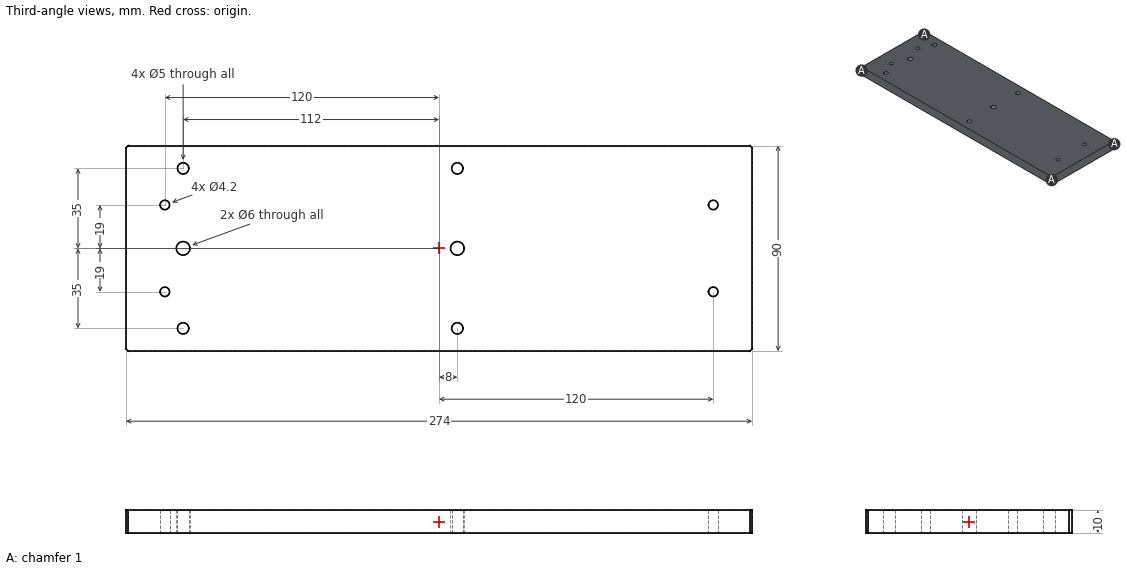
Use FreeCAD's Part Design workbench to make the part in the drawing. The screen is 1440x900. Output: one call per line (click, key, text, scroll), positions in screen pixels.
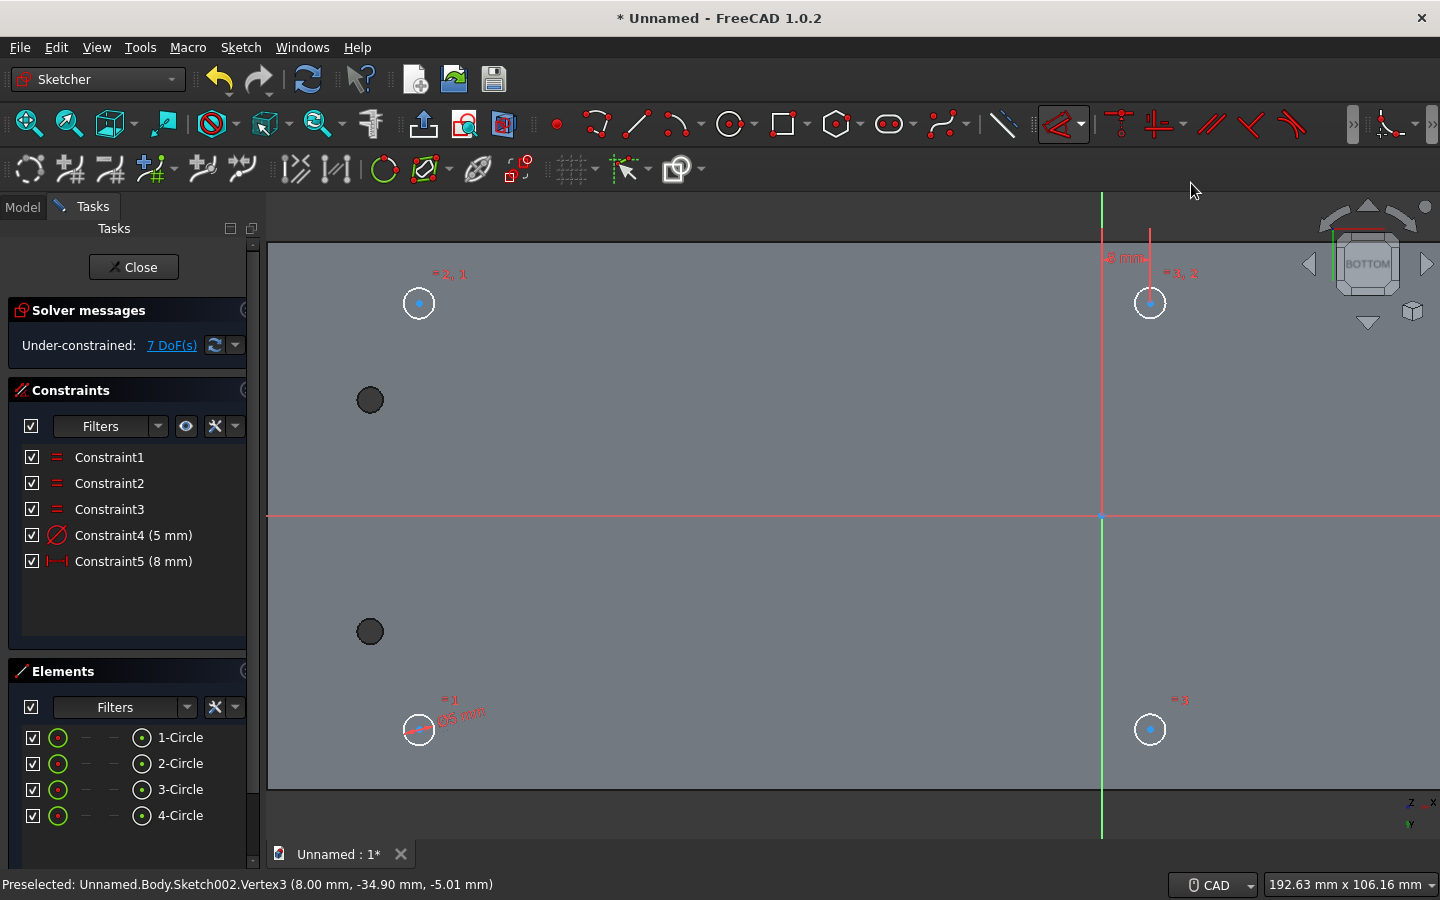
click(1150, 730)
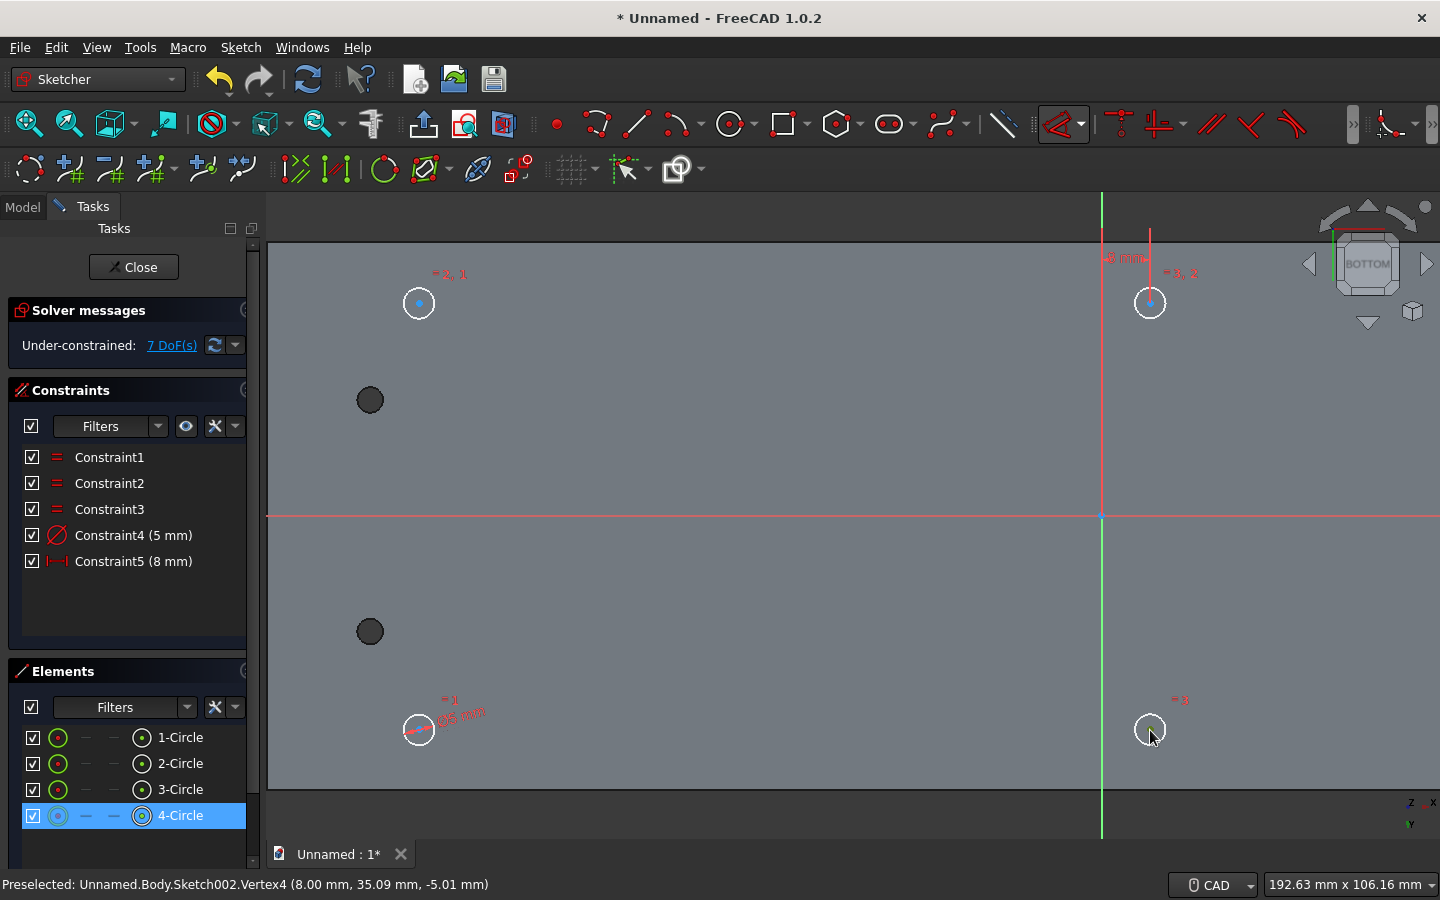
key(l)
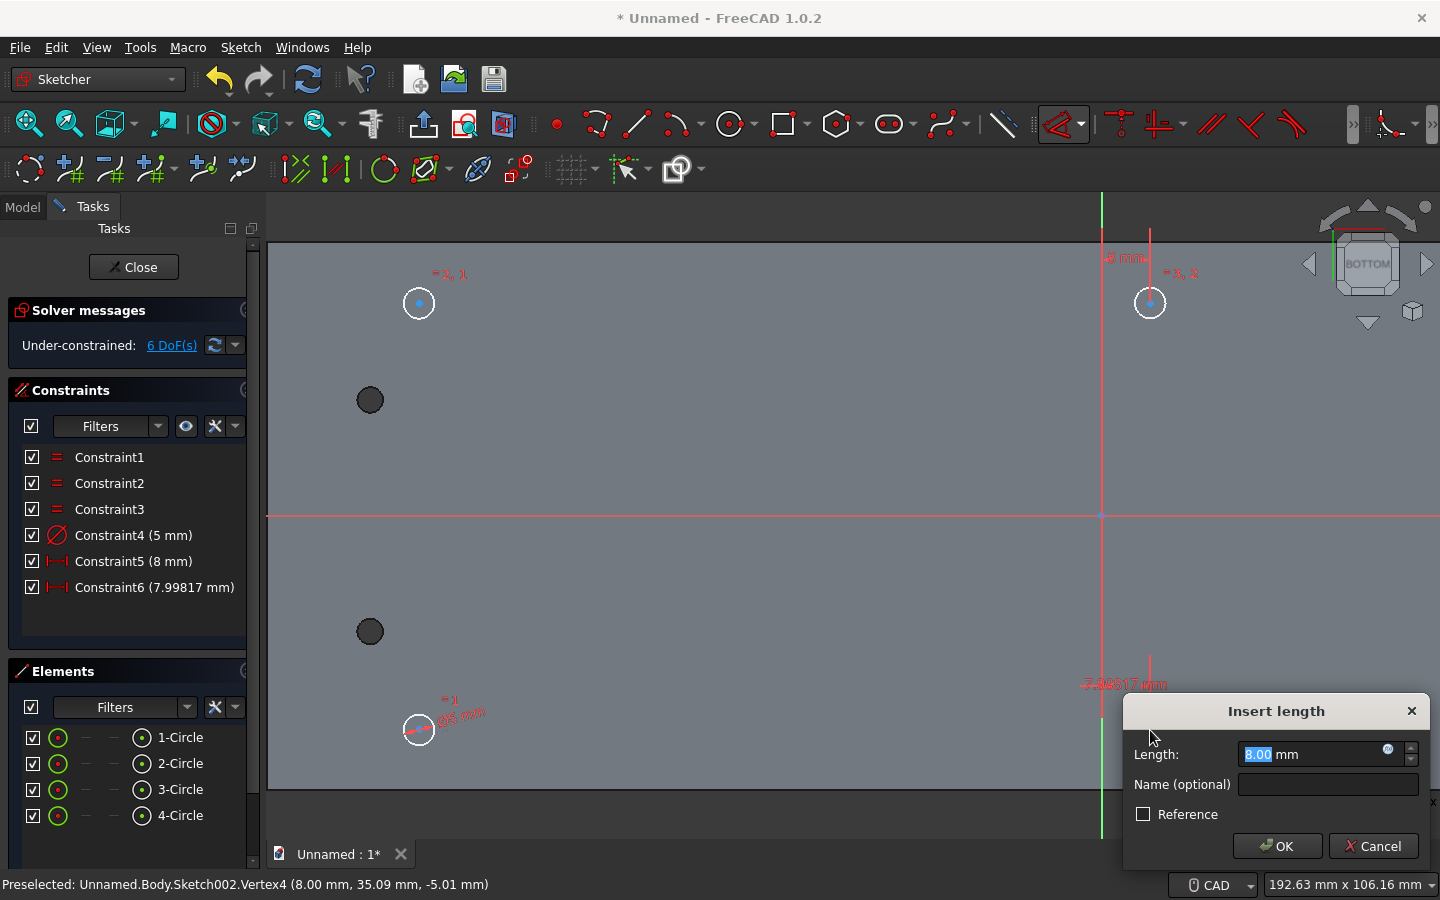
text(8)
key(Return)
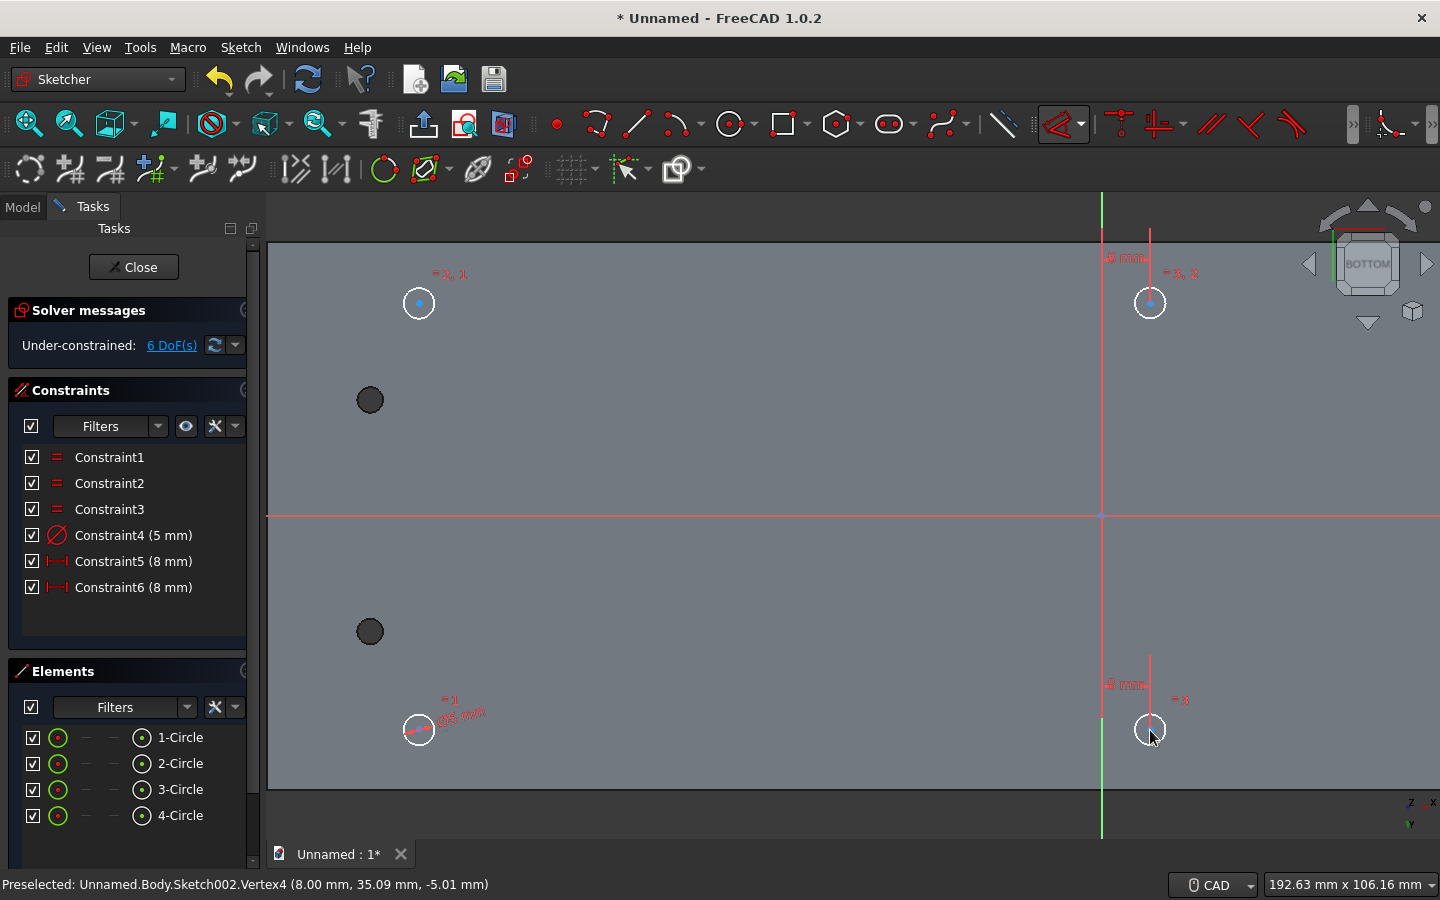
click(419, 730)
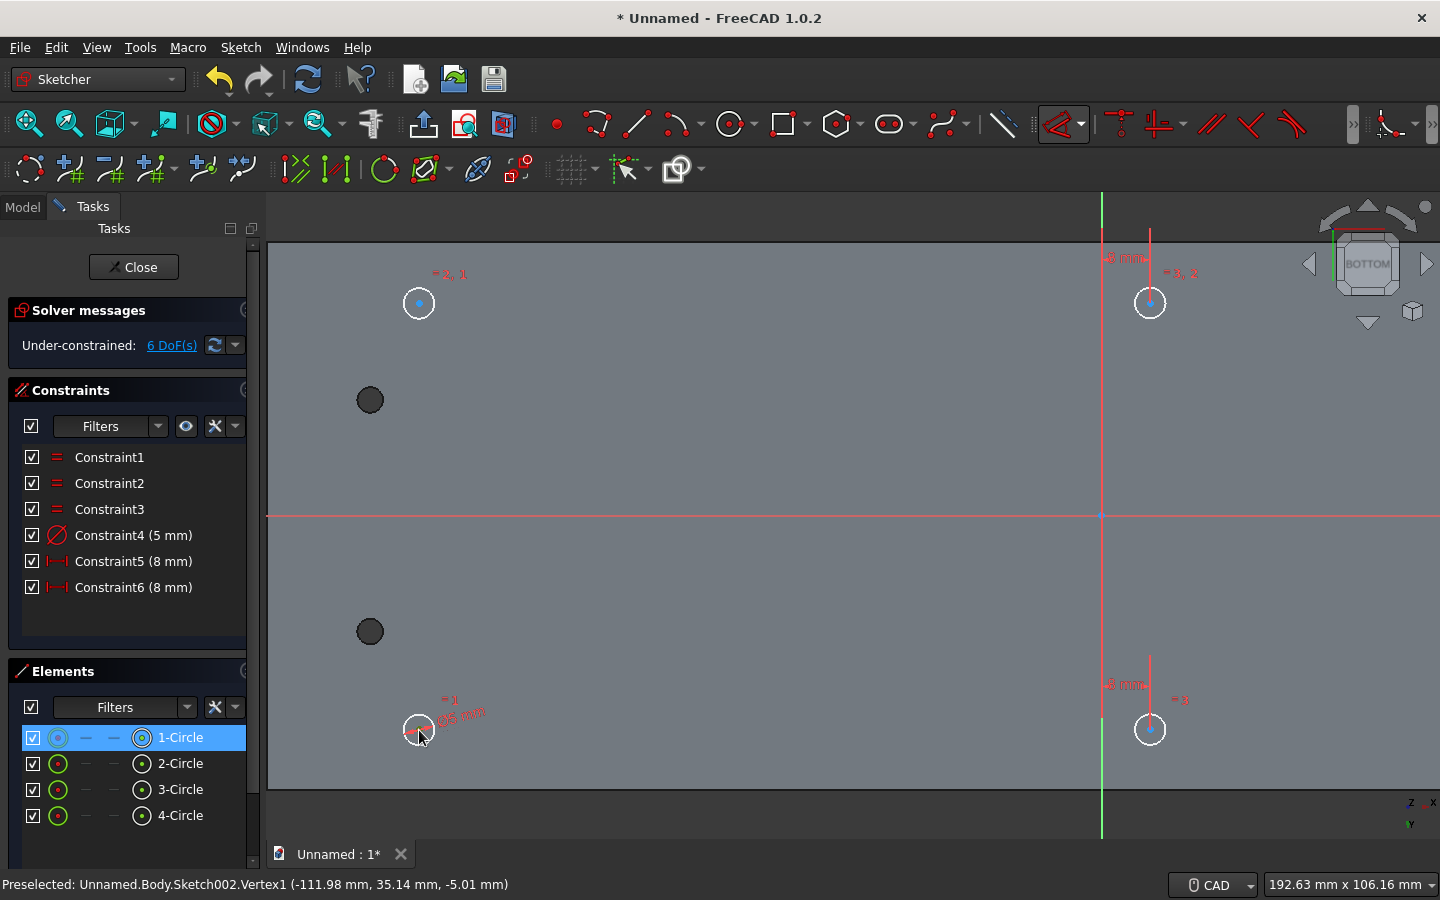
key(i)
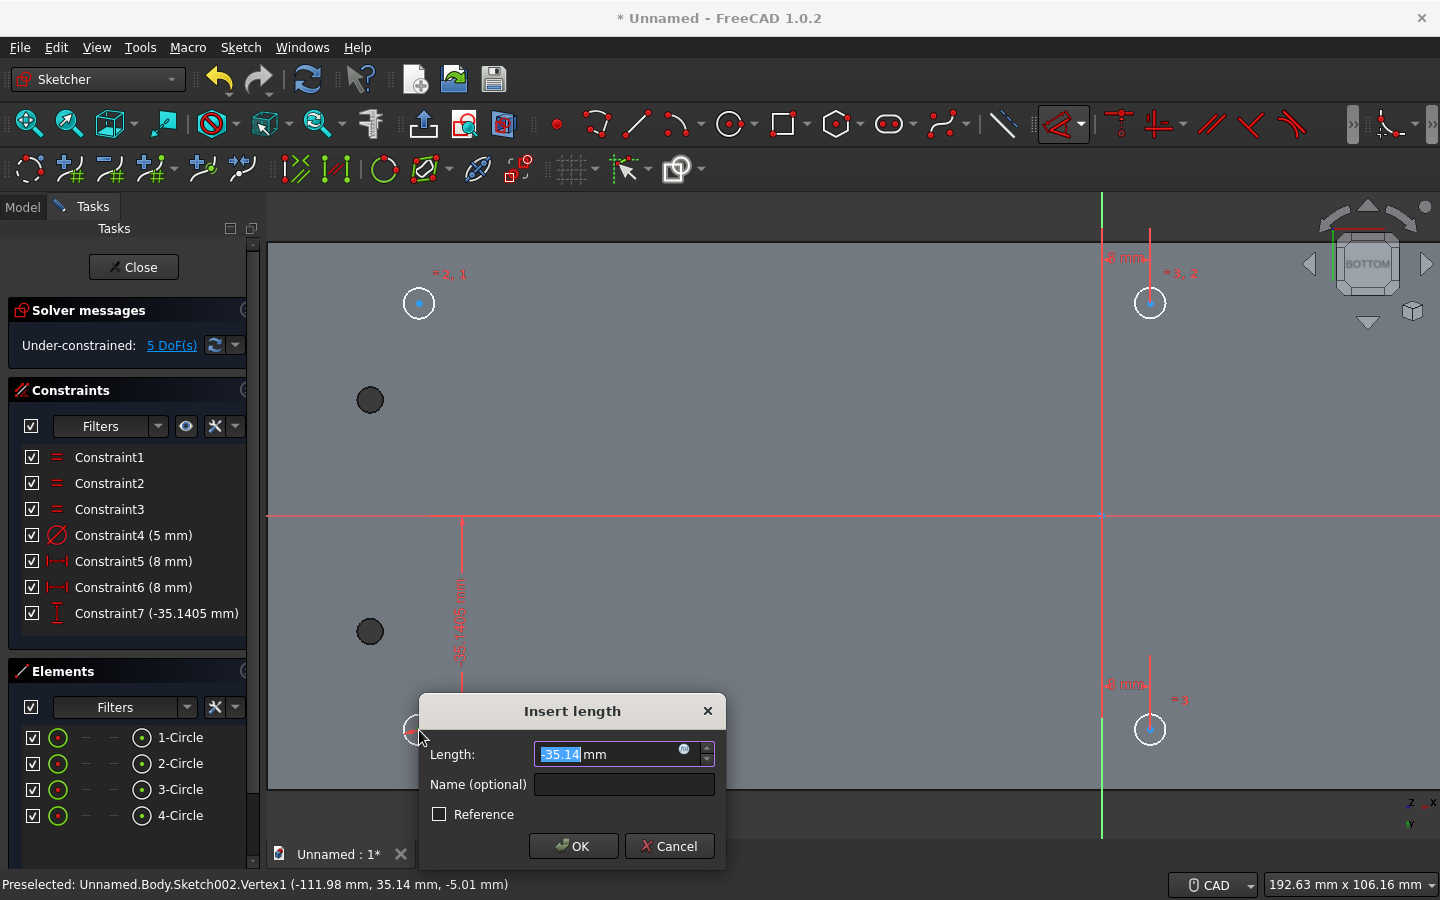
text(-35)
key(Return)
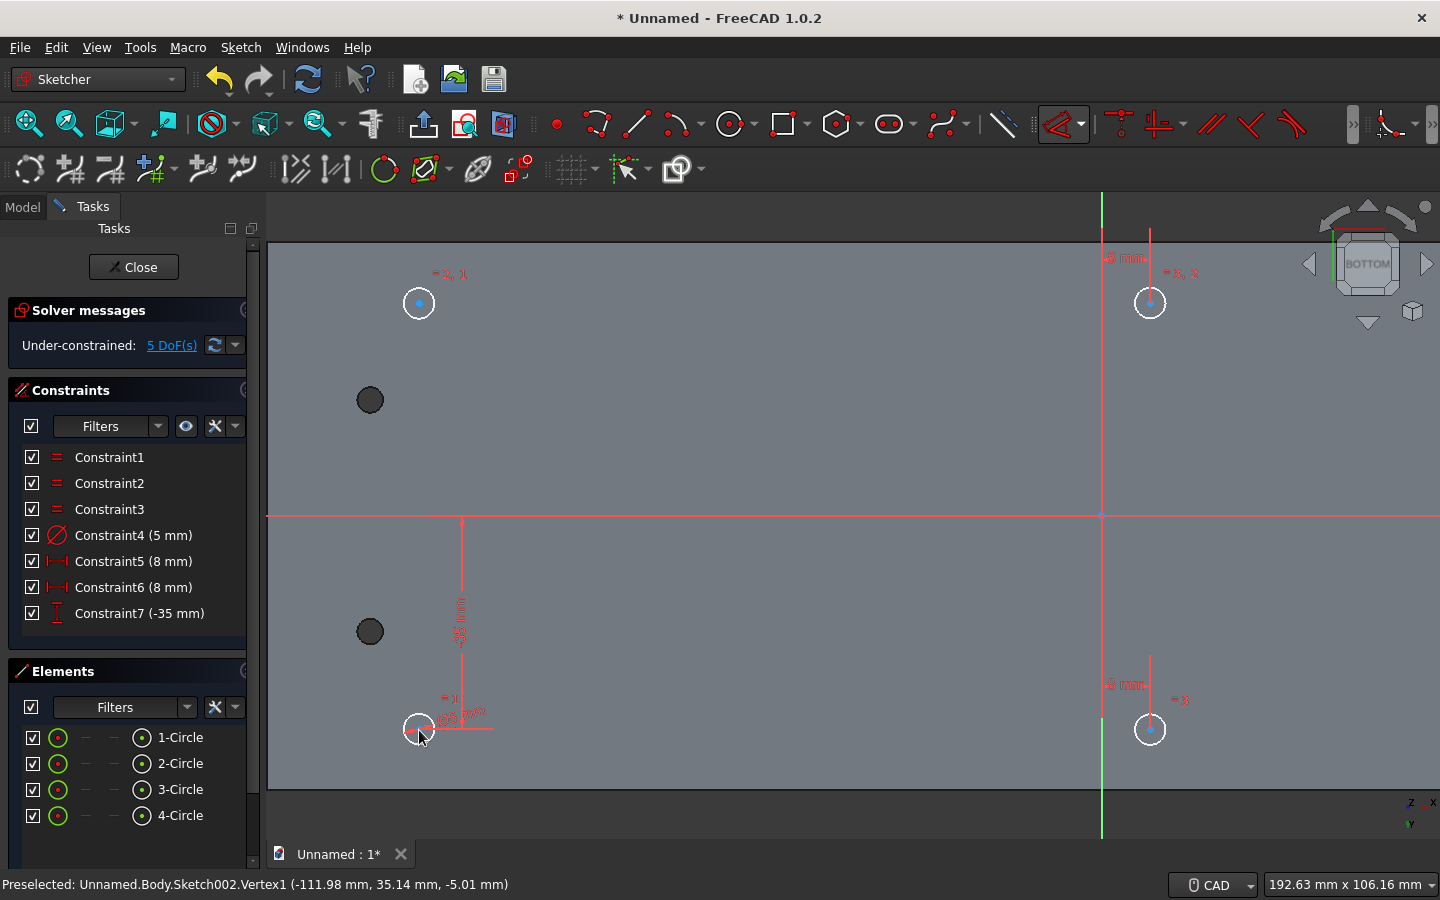
click(419, 303)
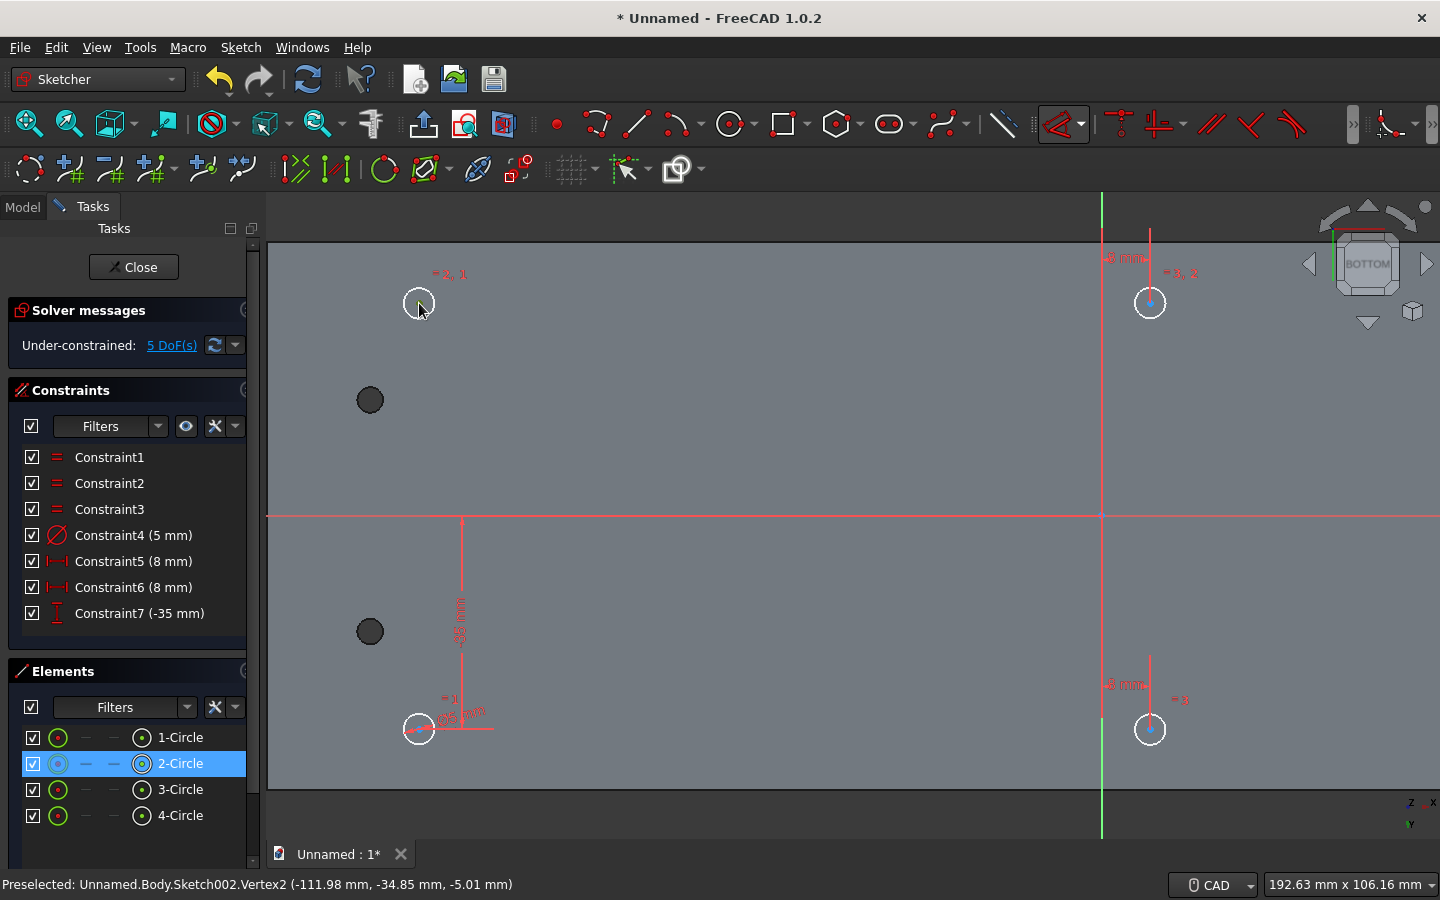
click(1084, 124)